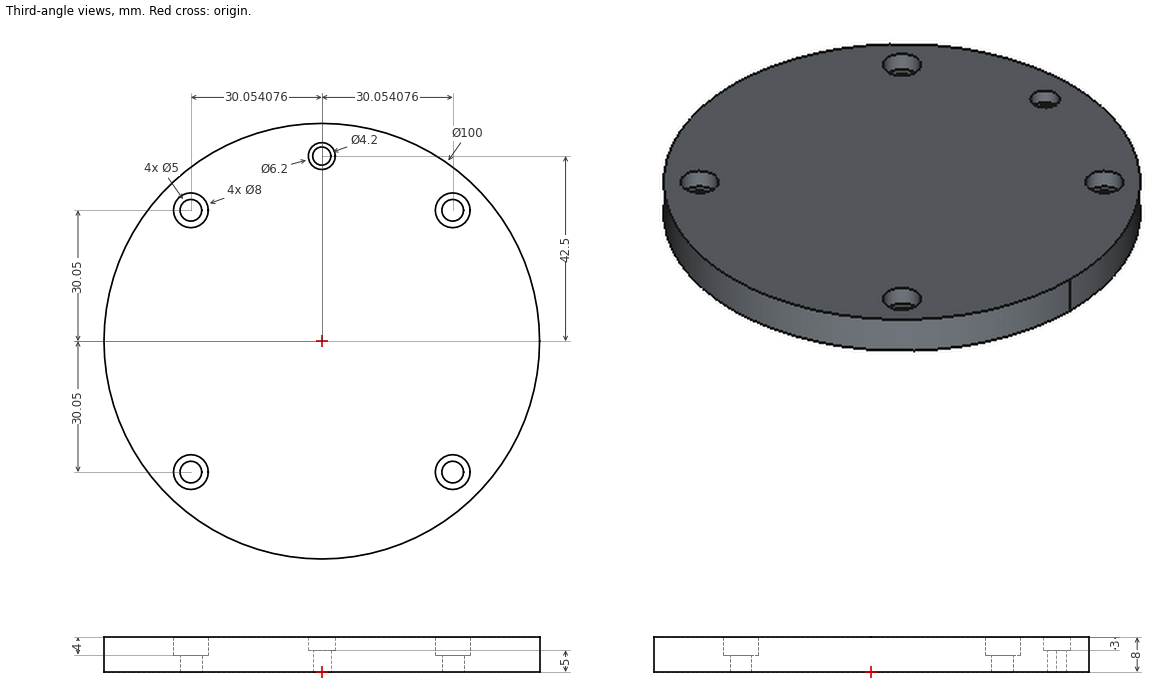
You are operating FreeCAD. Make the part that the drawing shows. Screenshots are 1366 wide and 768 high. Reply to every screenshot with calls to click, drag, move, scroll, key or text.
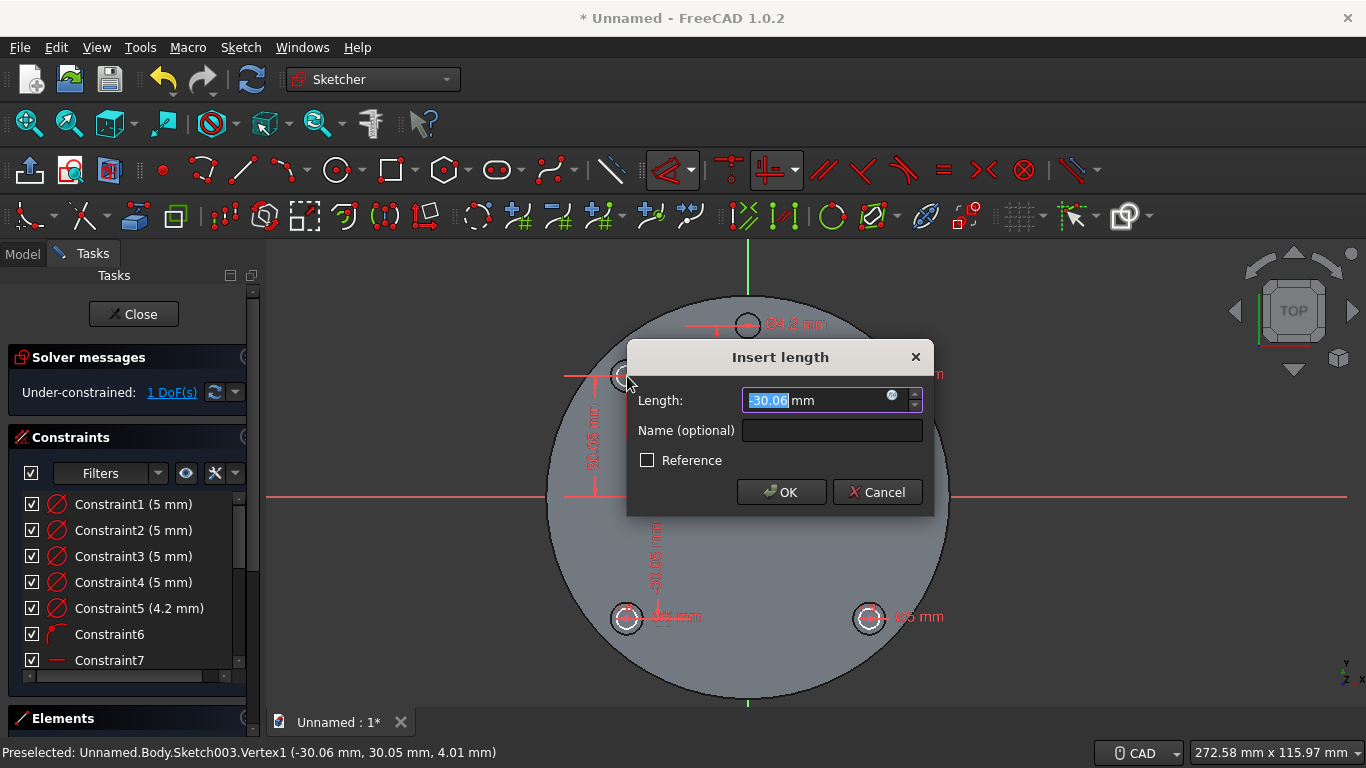
text(-30.054076)
key(Return)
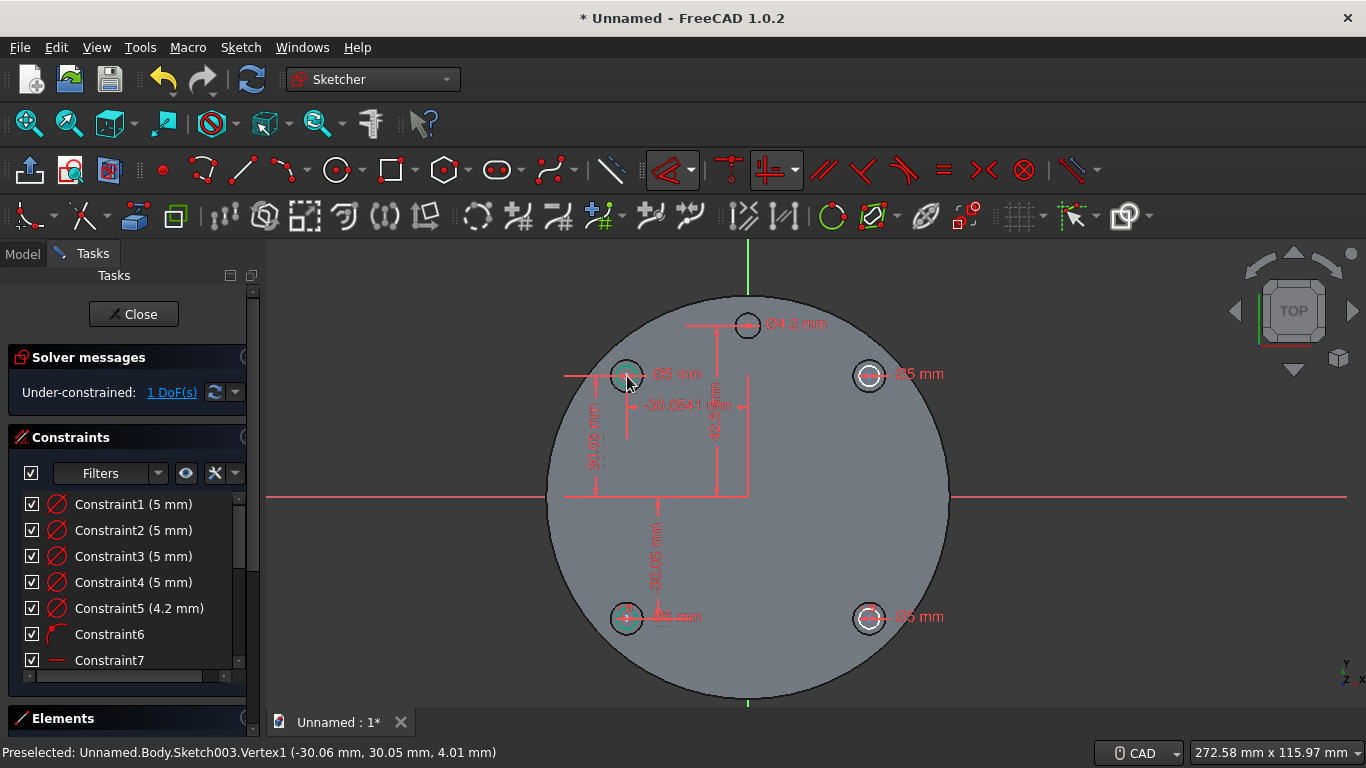
click(869, 376)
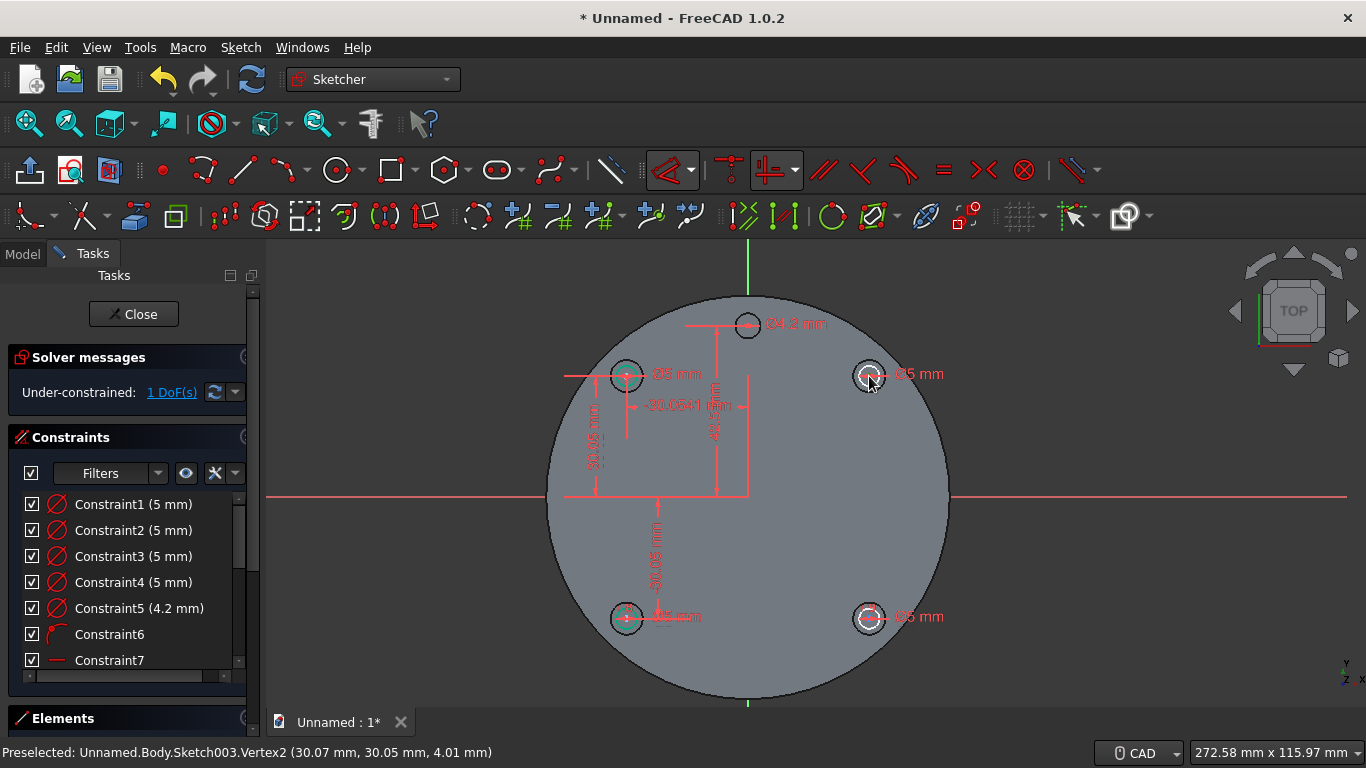
key(l)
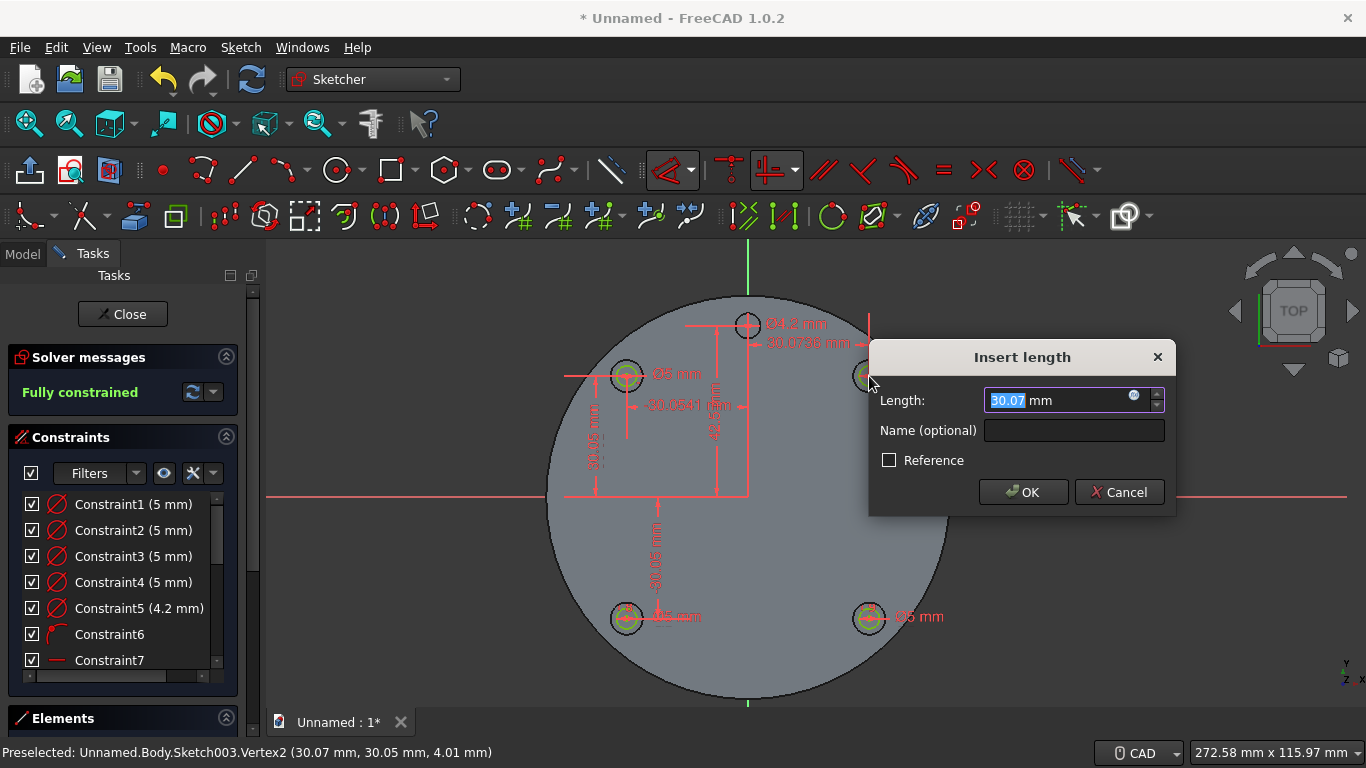
text(30.054076)
key(Return)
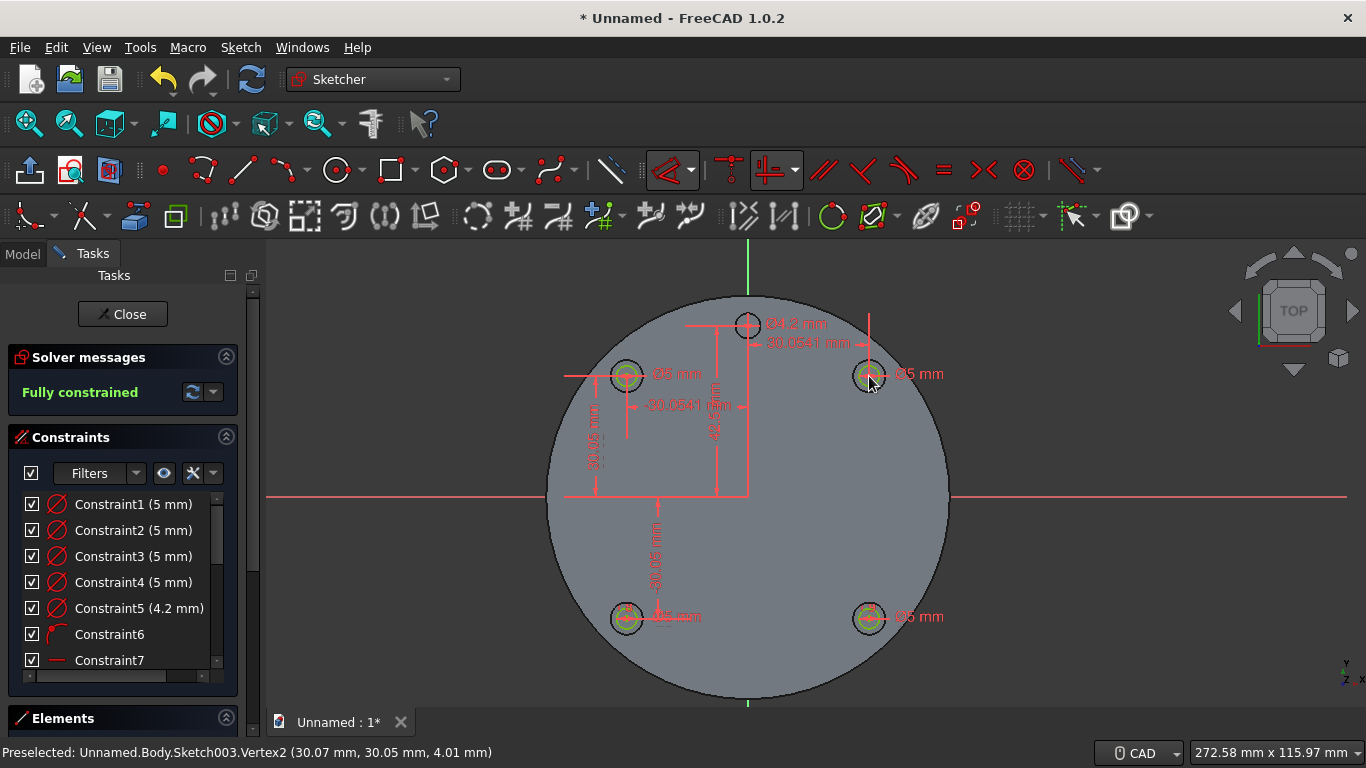
click(123, 314)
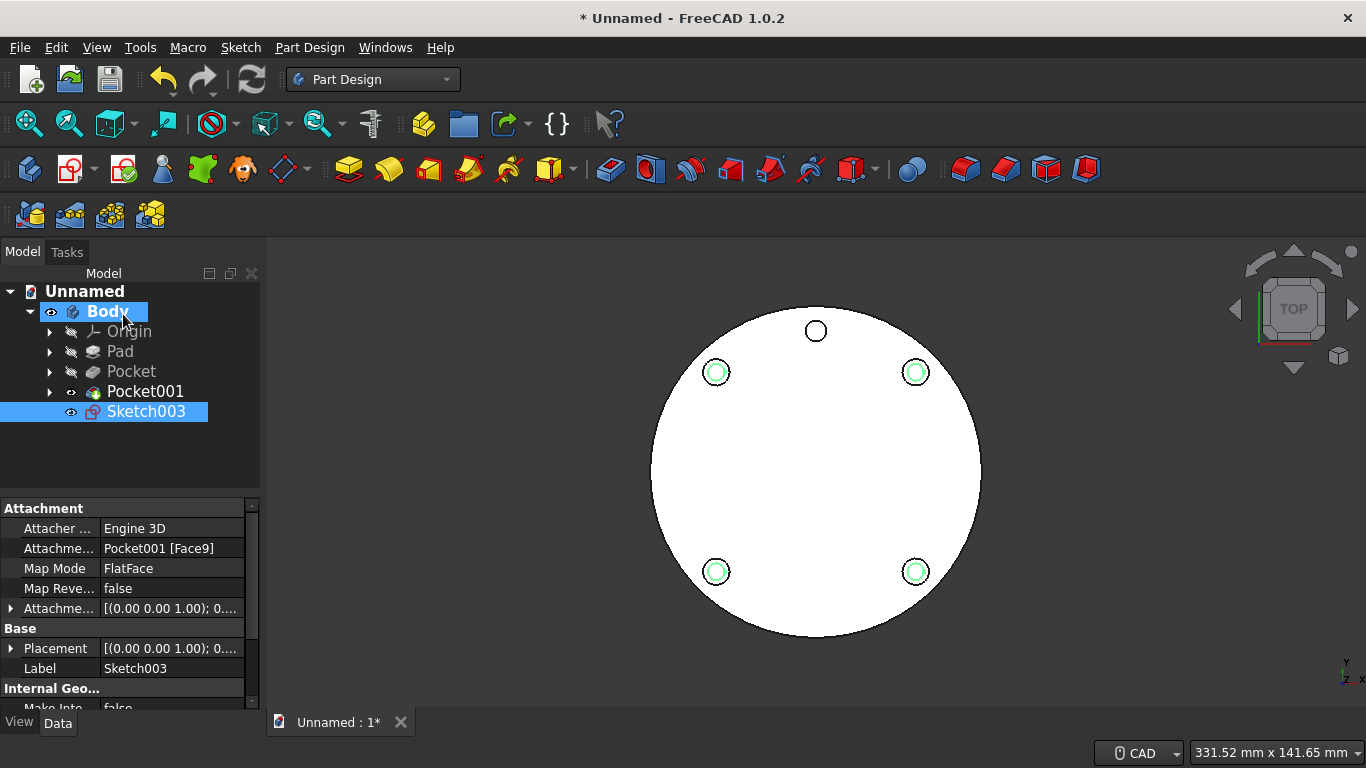
click(612, 170)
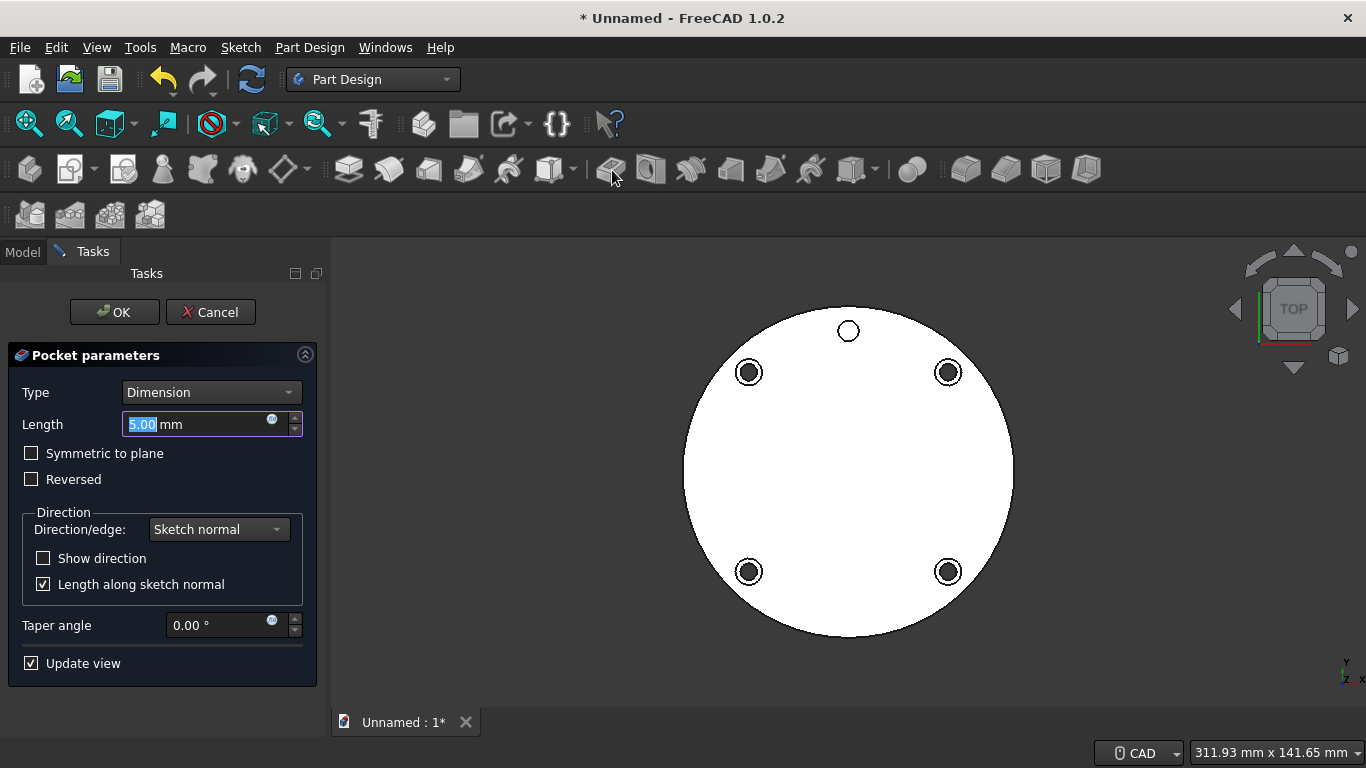
click(212, 392)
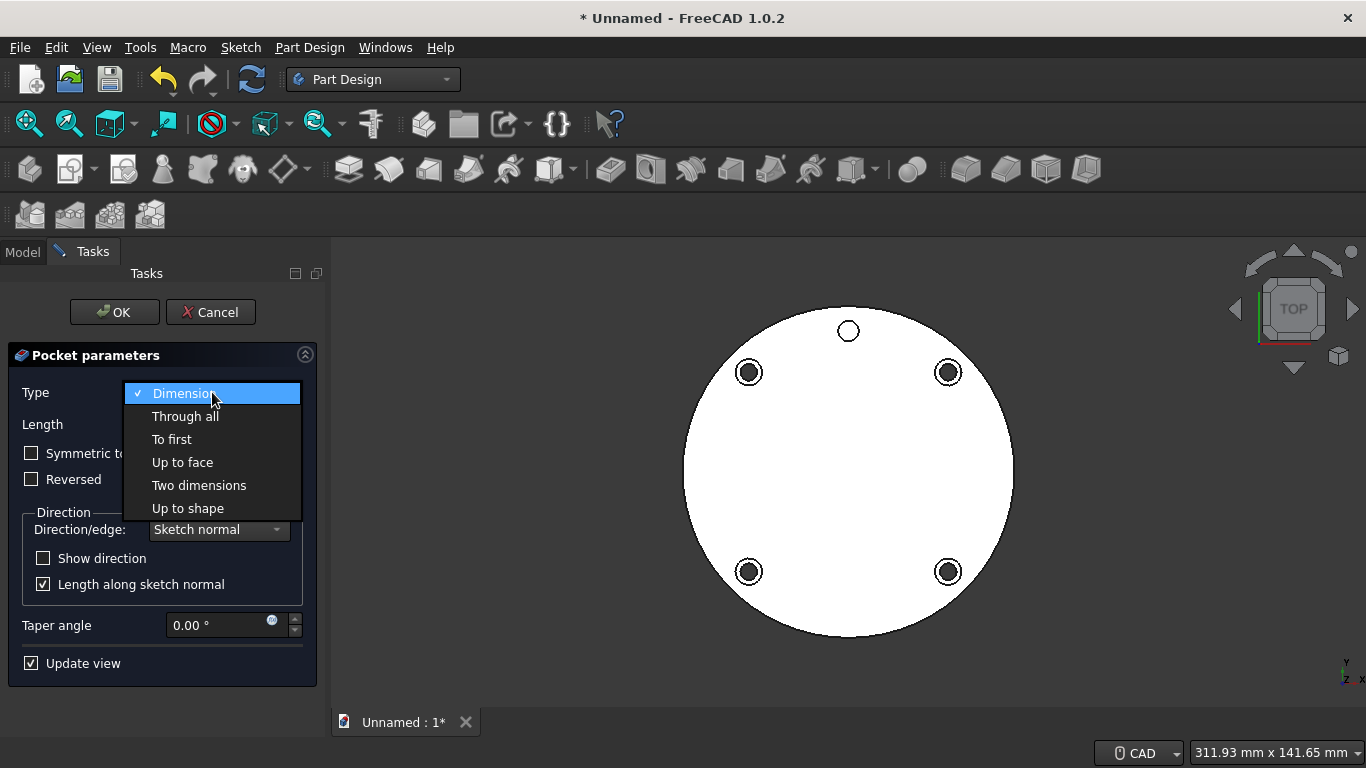
click(212, 416)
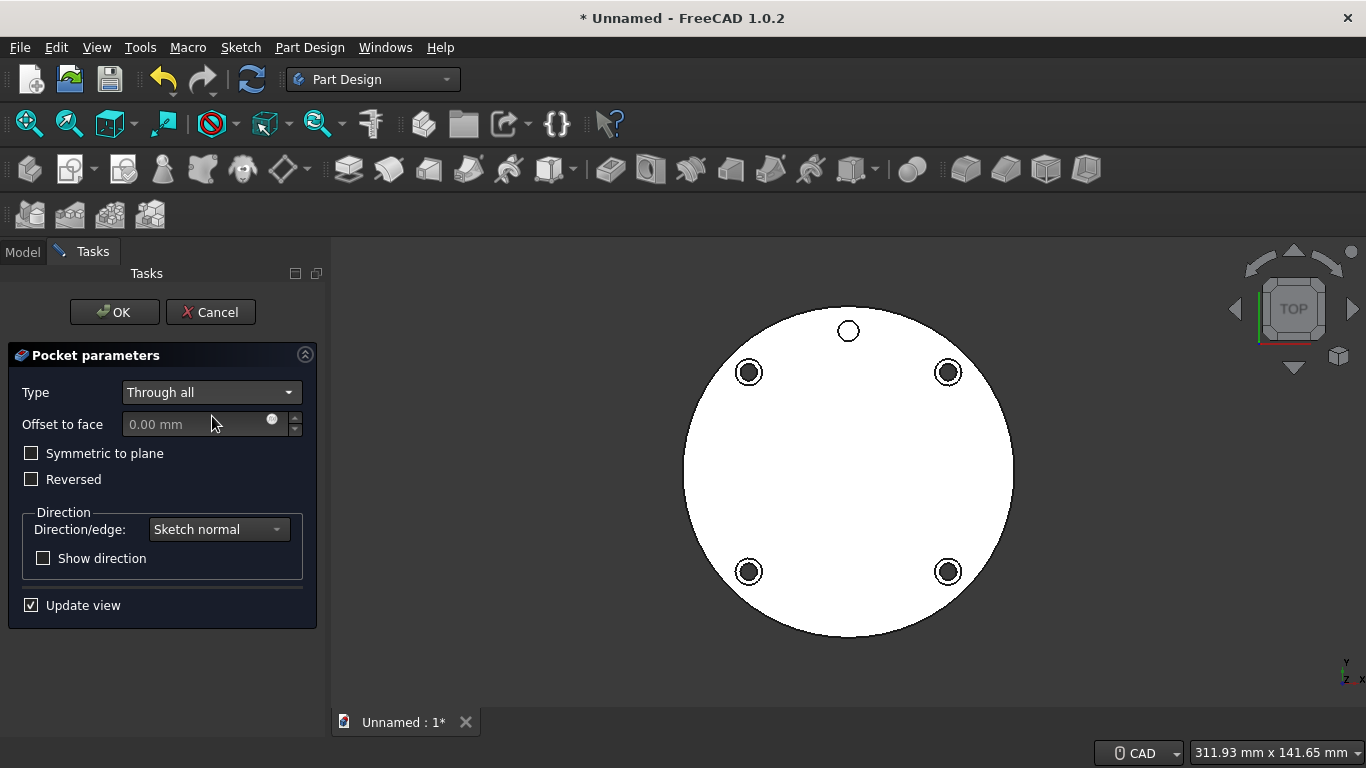
click(115, 312)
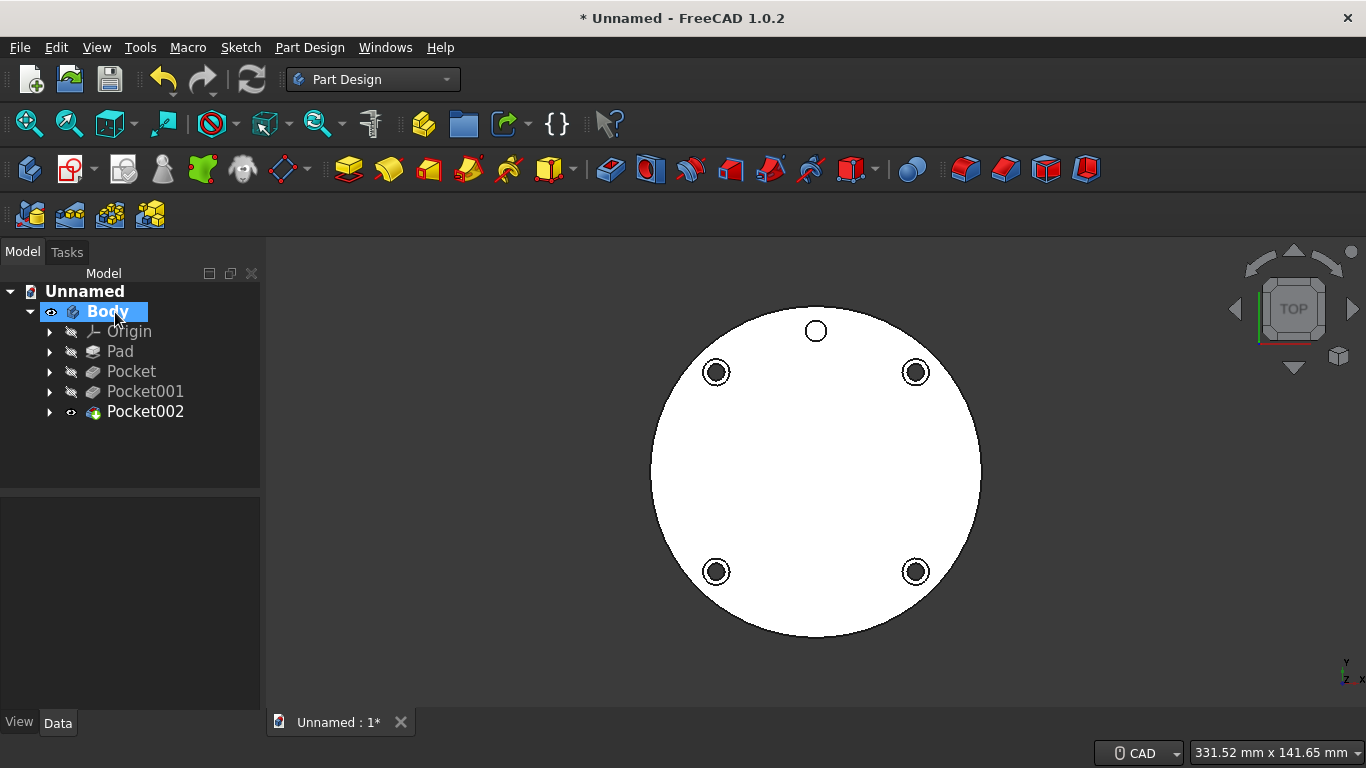
click(816, 330)